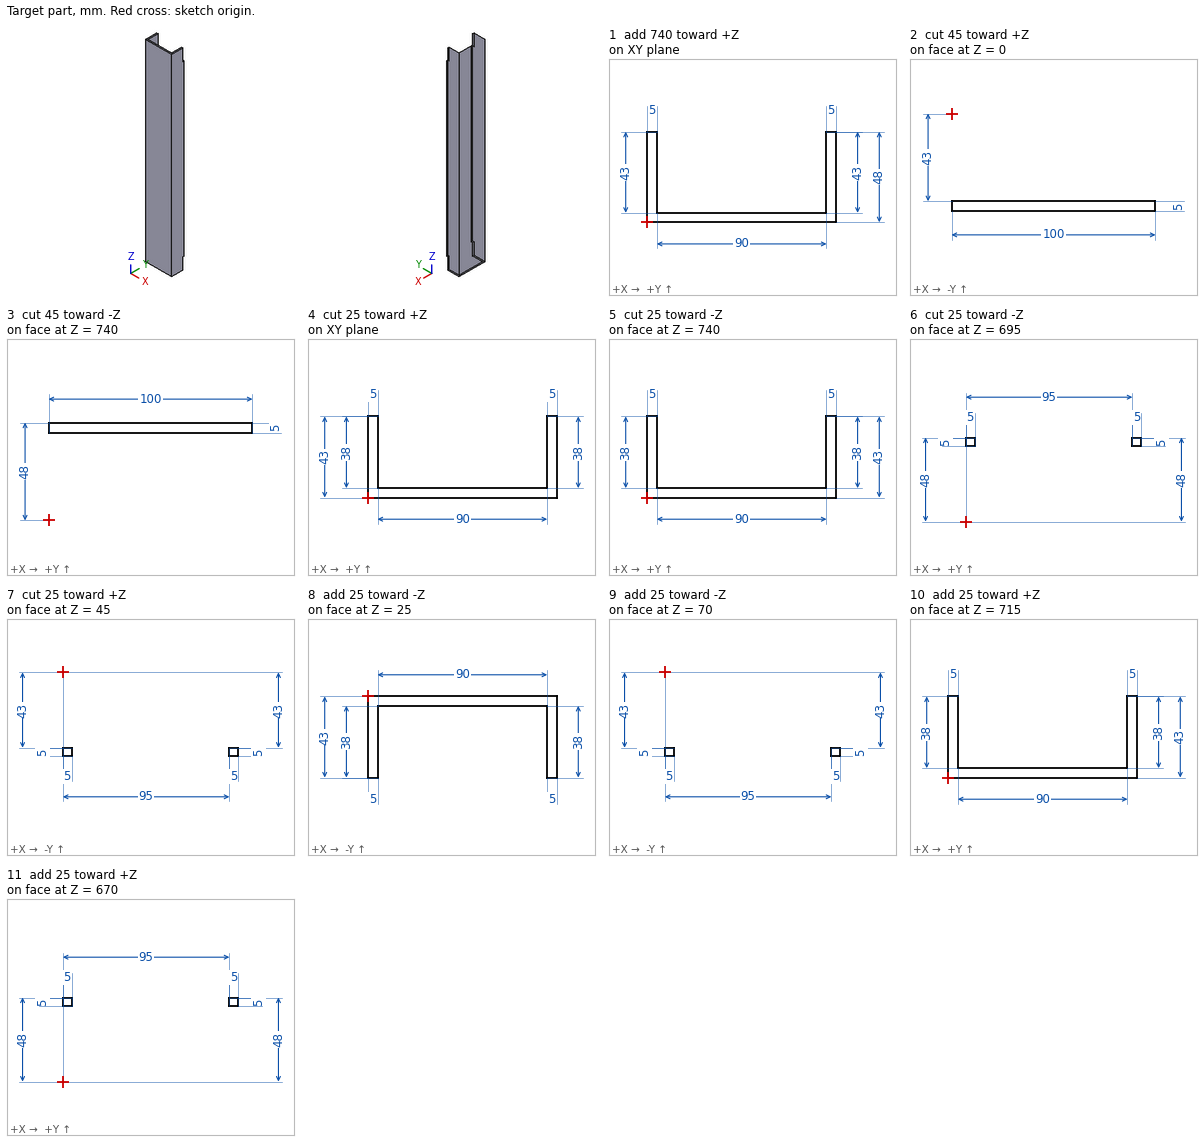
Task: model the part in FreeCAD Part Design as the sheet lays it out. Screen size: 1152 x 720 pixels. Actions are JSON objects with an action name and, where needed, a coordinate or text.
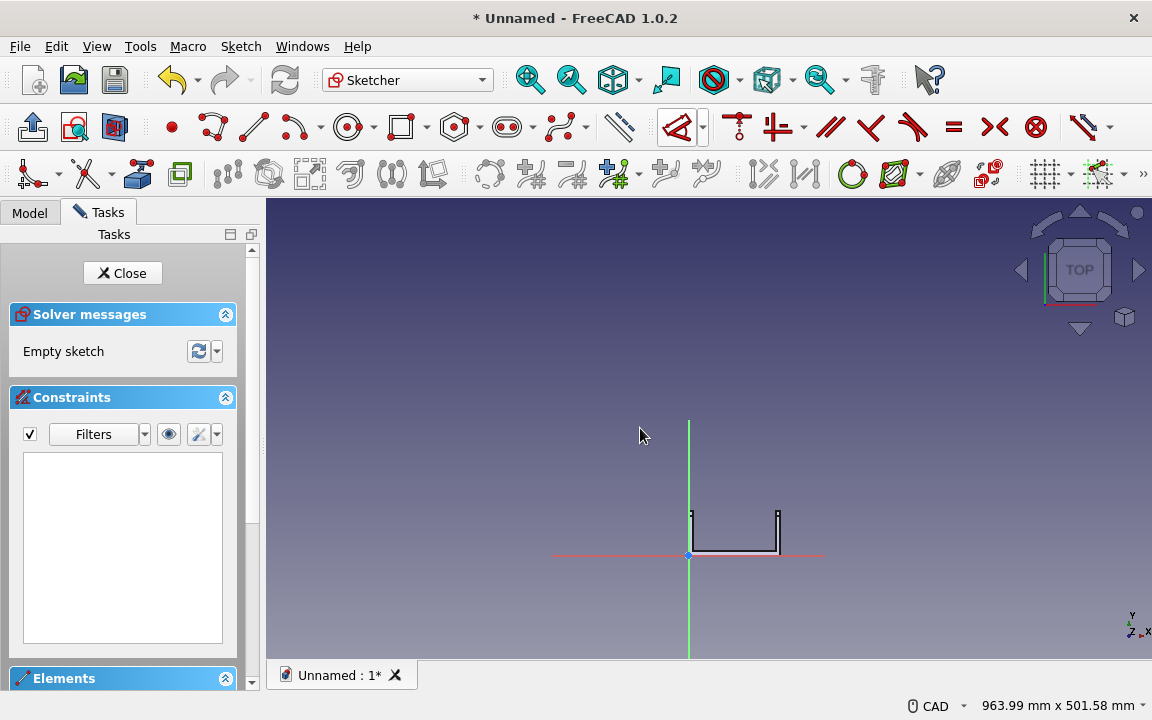
{"action": "scroll", "coordinate": [758, 563], "scroll_direction": "up", "scroll_amount": 8}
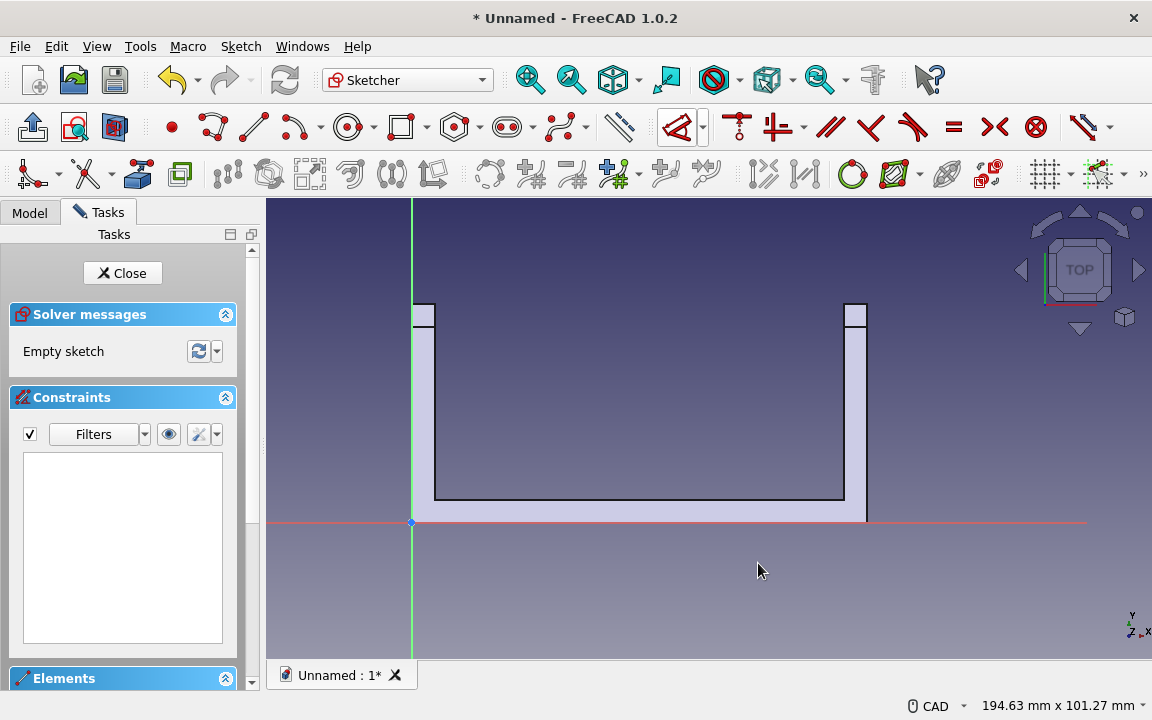
{"action": "key", "text": "g m"}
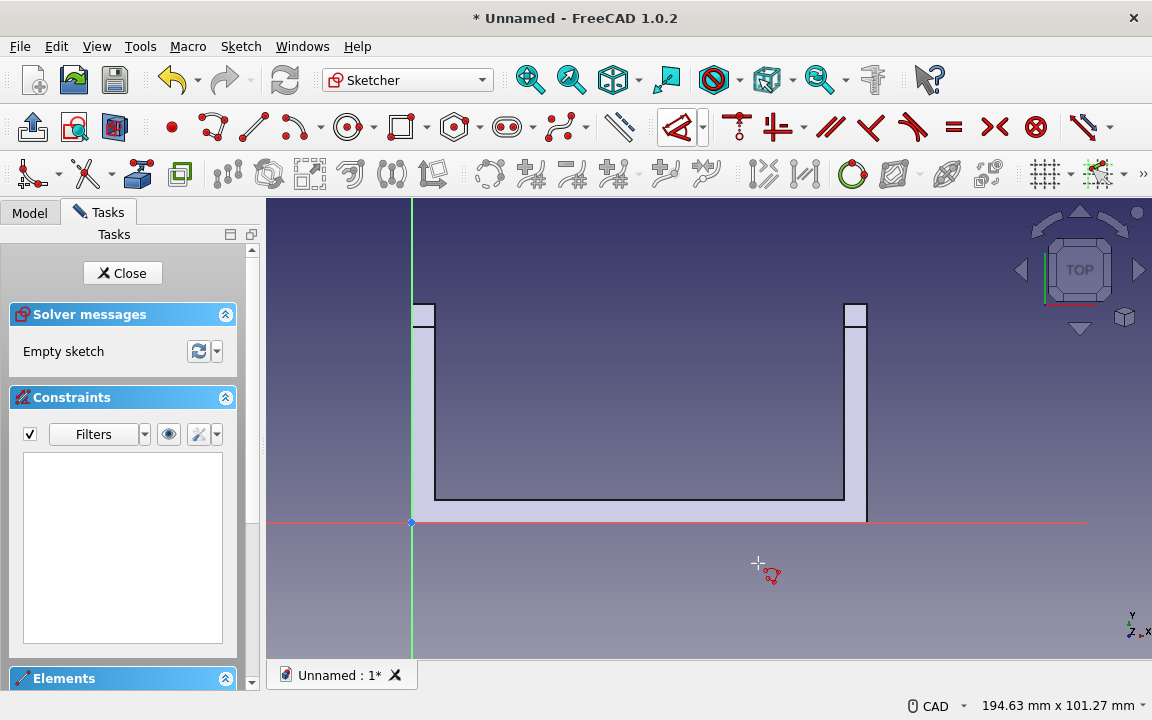
{"action": "left_click", "coordinate": [412, 523]}
{"action": "left_click", "coordinate": [867, 514]}
{"action": "left_click", "coordinate": [867, 327]}
{"action": "left_click", "coordinate": [844, 327]}
{"action": "left_click", "coordinate": [844, 500]}
{"action": "left_click", "coordinate": [435, 500]}
{"action": "left_click", "coordinate": [435, 327]}
{"action": "left_click", "coordinate": [421, 327]}
{"action": "left_click", "coordinate": [412, 523]}
{"action": "key", "text": "Escape"}
{"action": "key", "text": "Escape"}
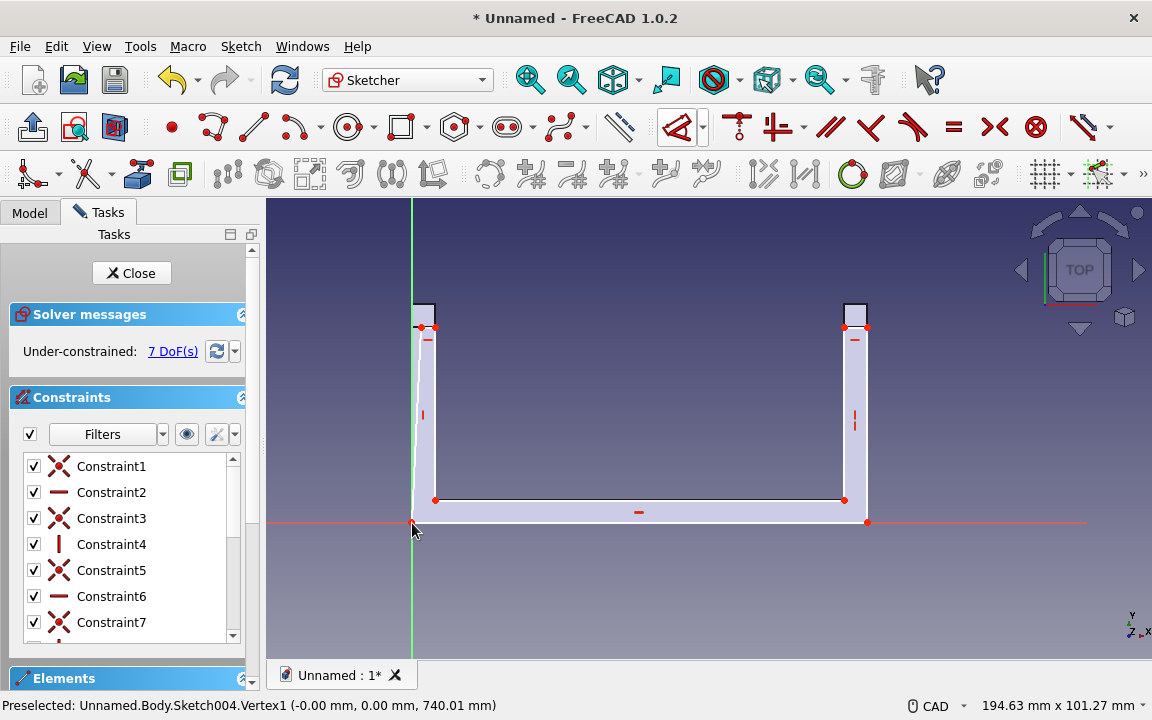
{"action": "left_click", "coordinate": [415, 464]}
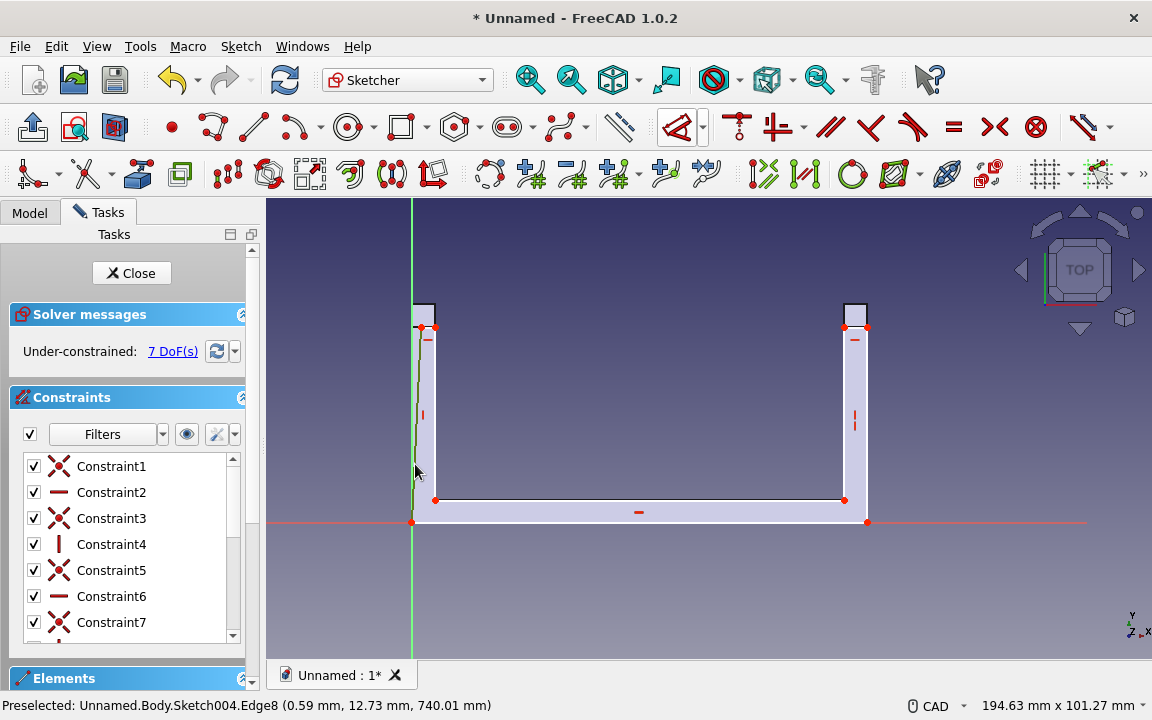
{"action": "key", "text": "v"}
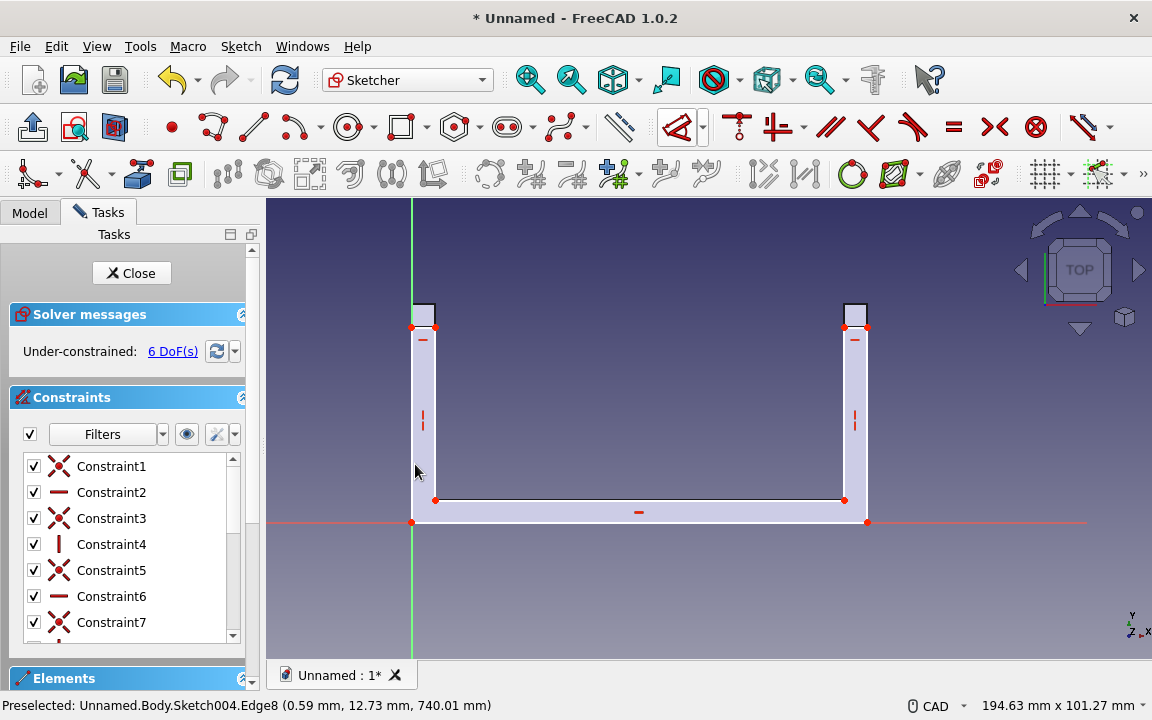
{"action": "scroll", "coordinate": [858, 328], "scroll_direction": "up", "scroll_amount": 3}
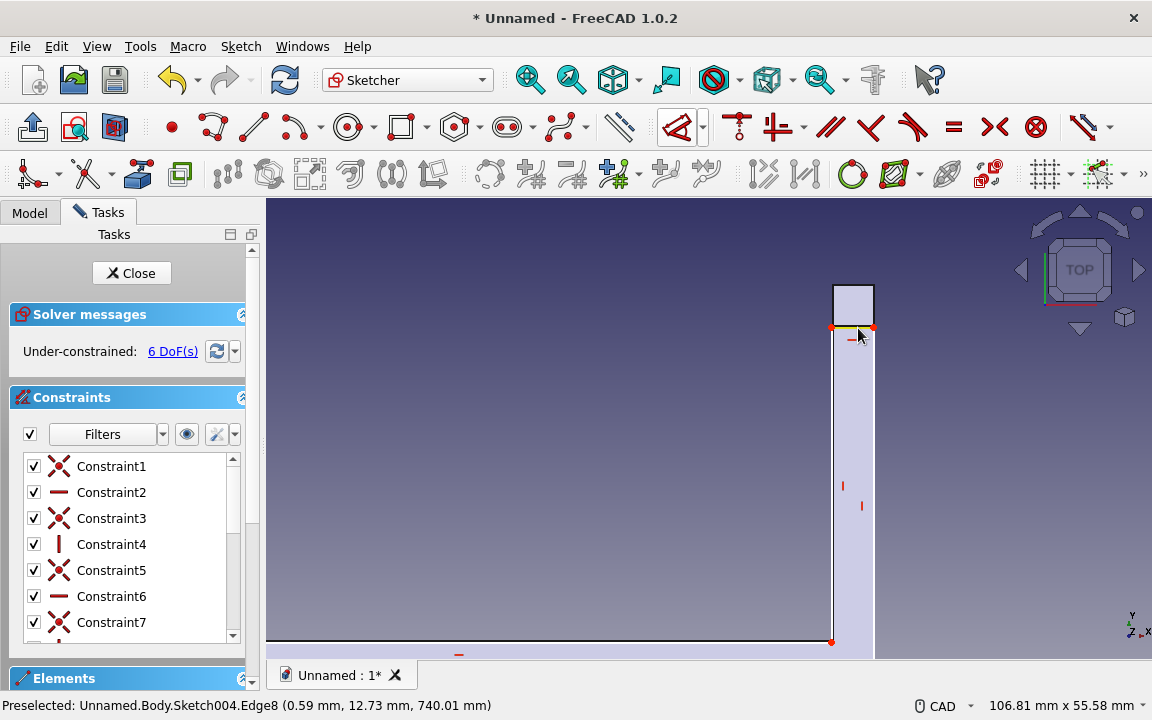
{"action": "left_click", "coordinate": [857, 328]}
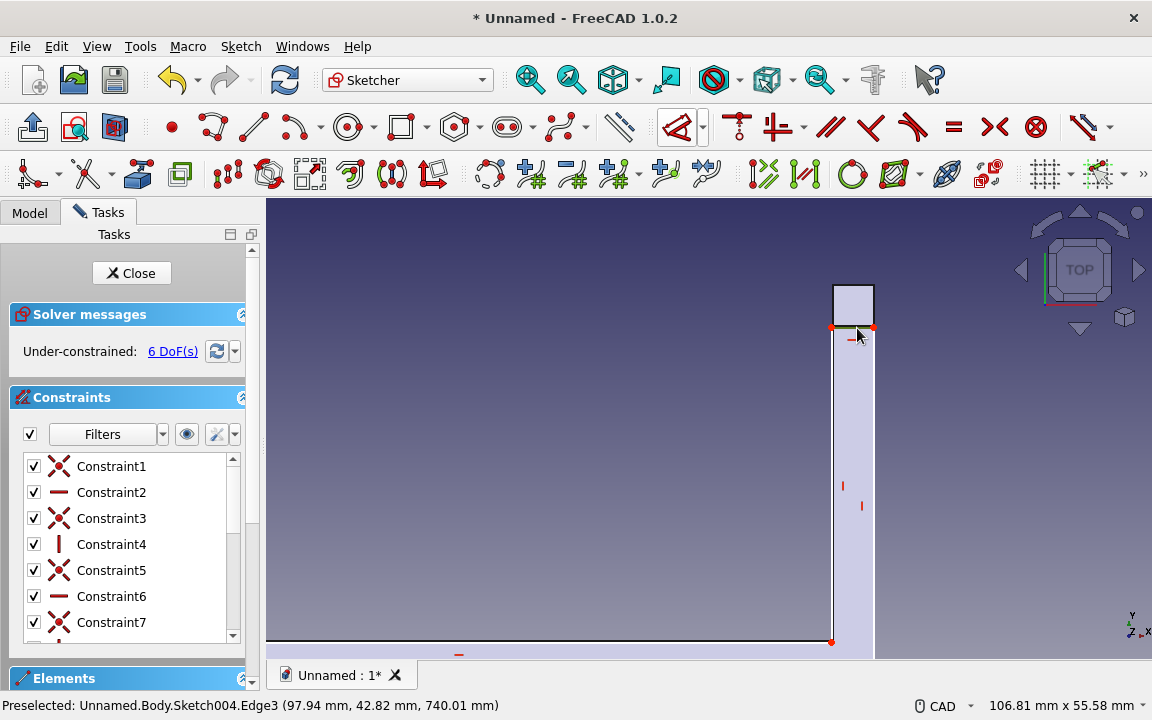
{"action": "key", "text": "l"}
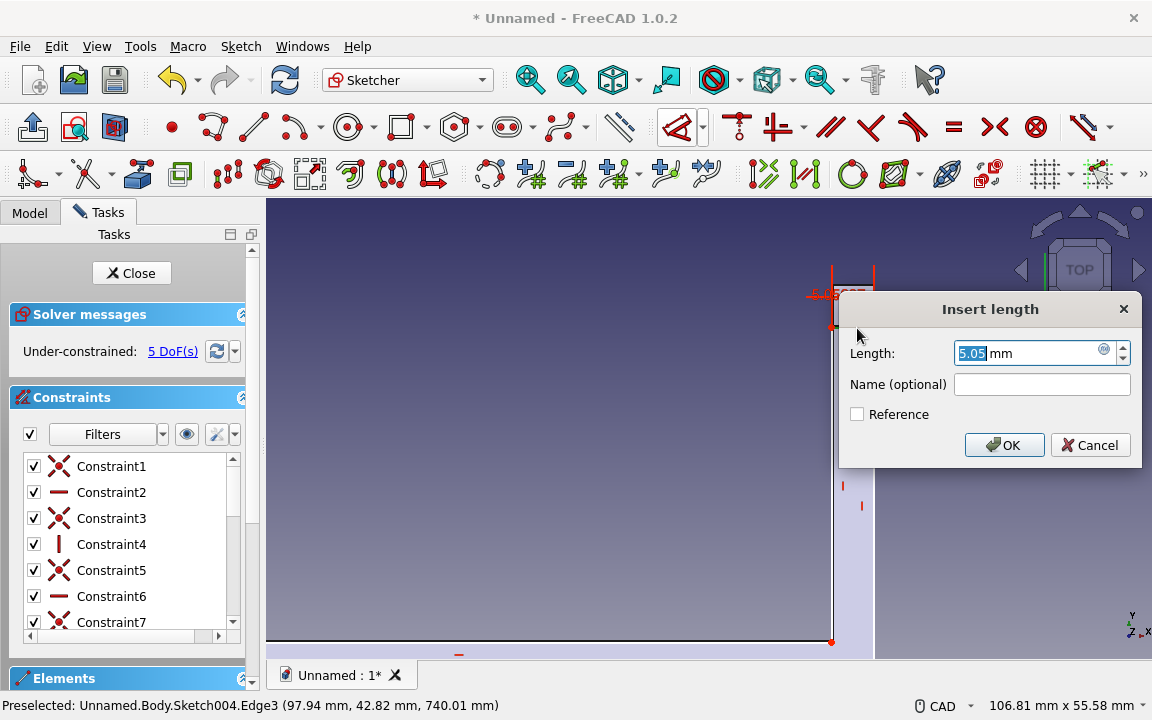
{"action": "type", "text": "5"}
{"action": "key", "text": "Return"}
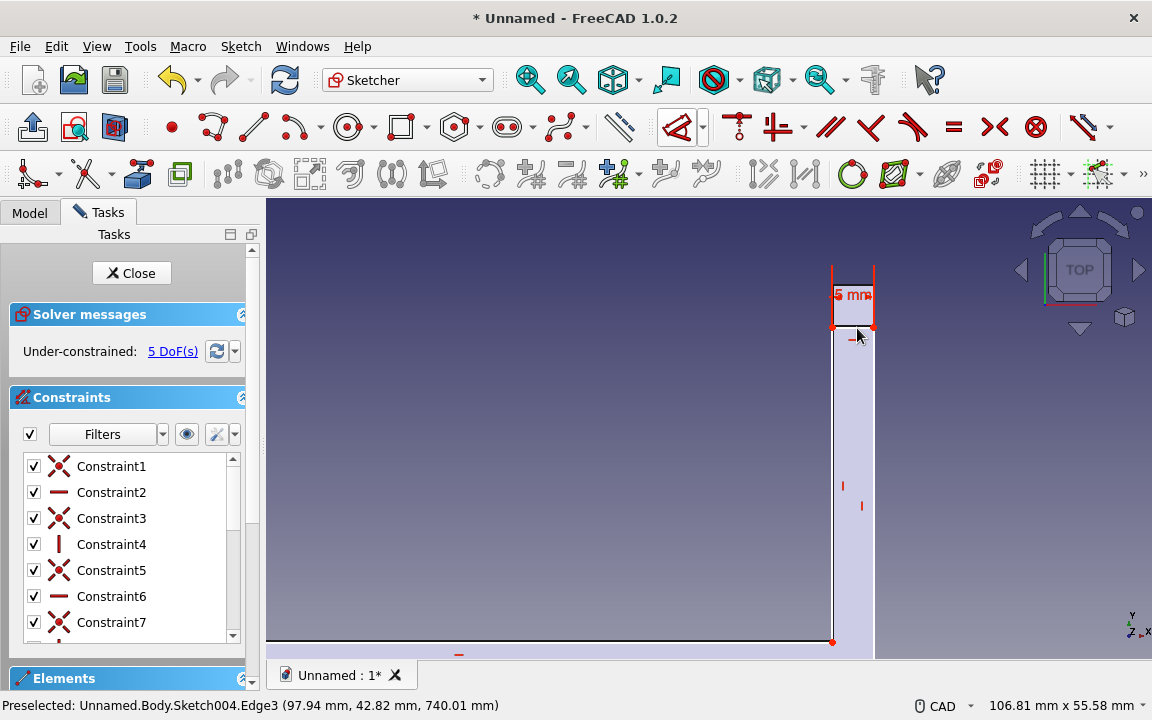
{"action": "scroll", "coordinate": [861, 336], "scroll_direction": "down", "scroll_amount": 3}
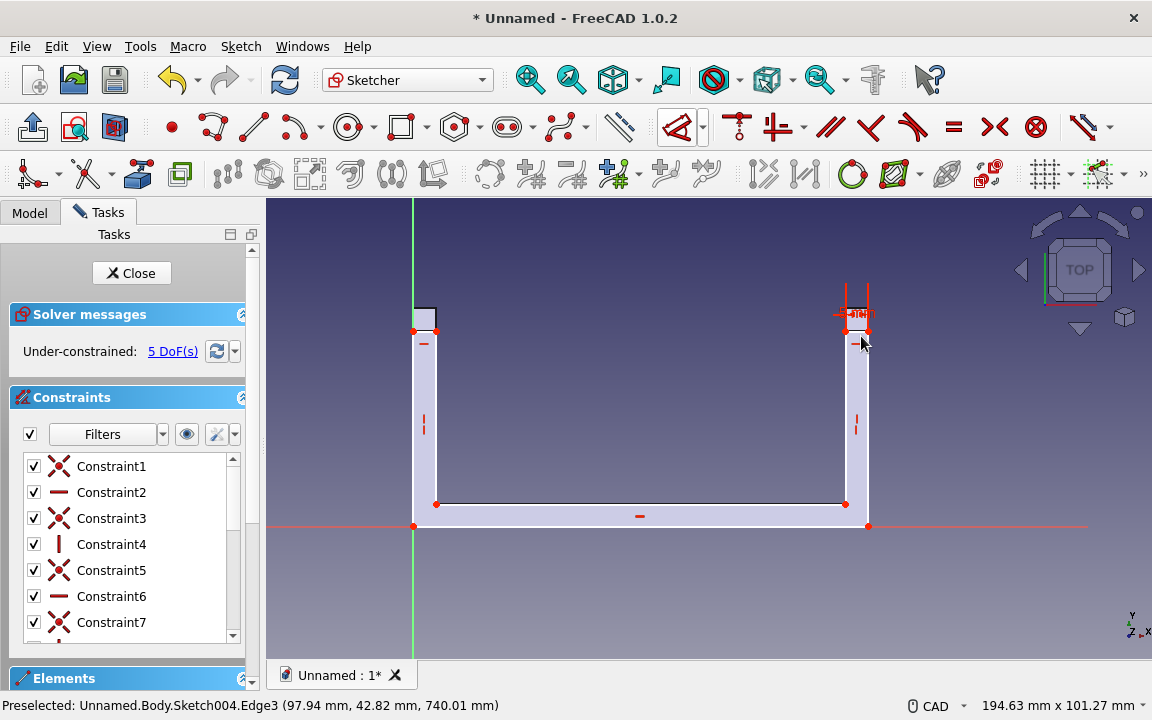
{"action": "scroll", "coordinate": [429, 332], "scroll_direction": "up", "scroll_amount": 4}